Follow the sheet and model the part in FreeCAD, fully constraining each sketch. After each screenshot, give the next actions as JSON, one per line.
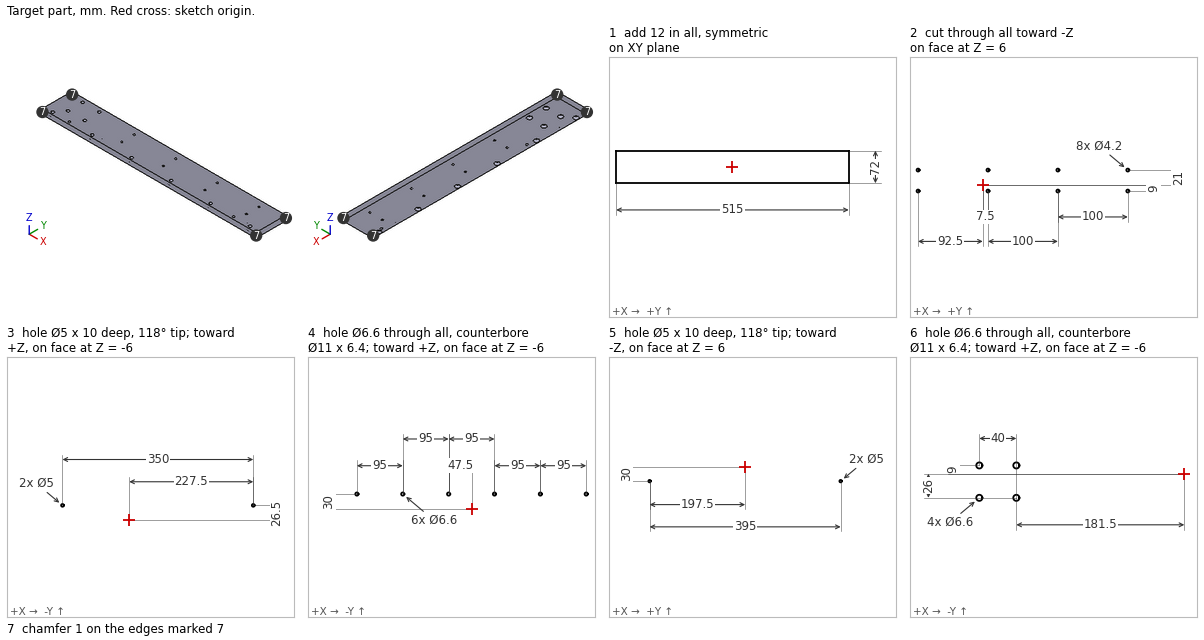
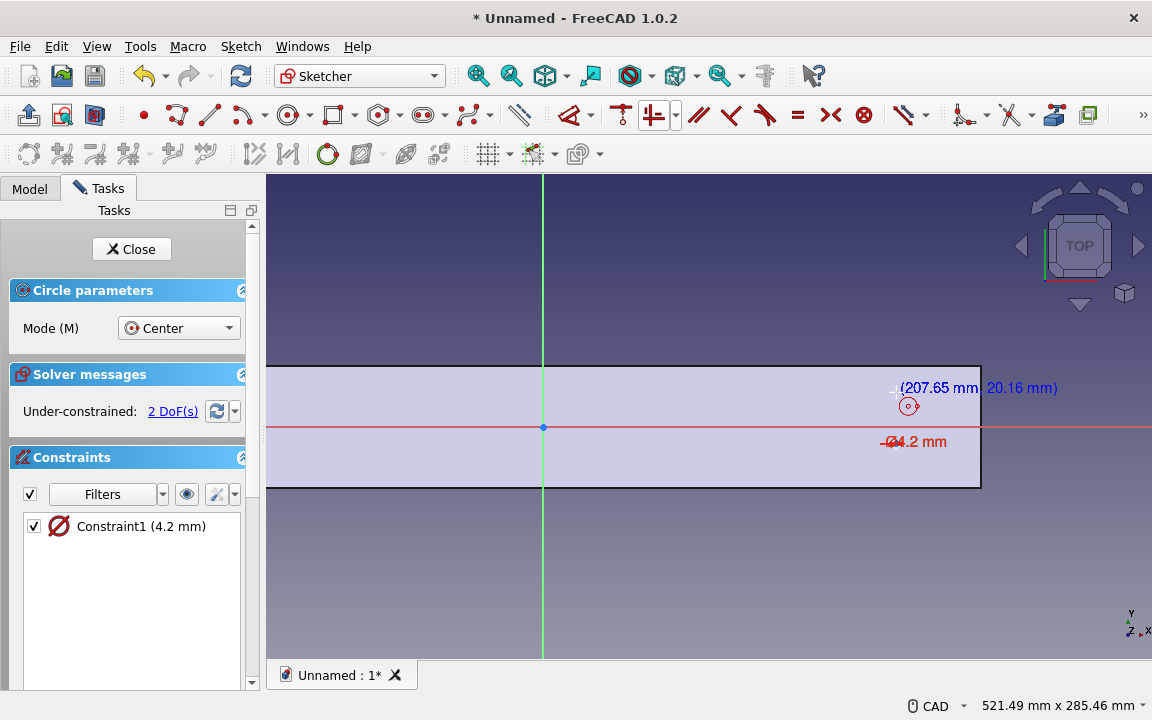
{"action": "left_click", "coordinate": [896, 392]}
{"action": "mouse_move", "coordinate": [898, 389]}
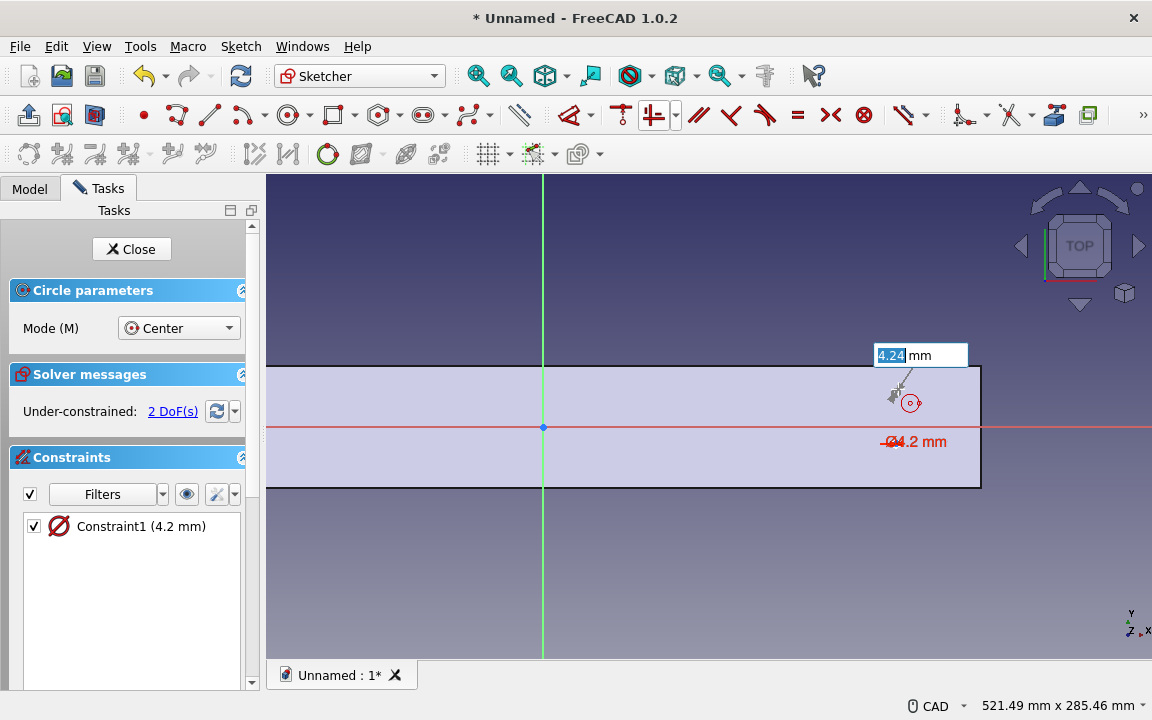
{"action": "type", "text": "4.2"}
{"action": "key", "text": "Return"}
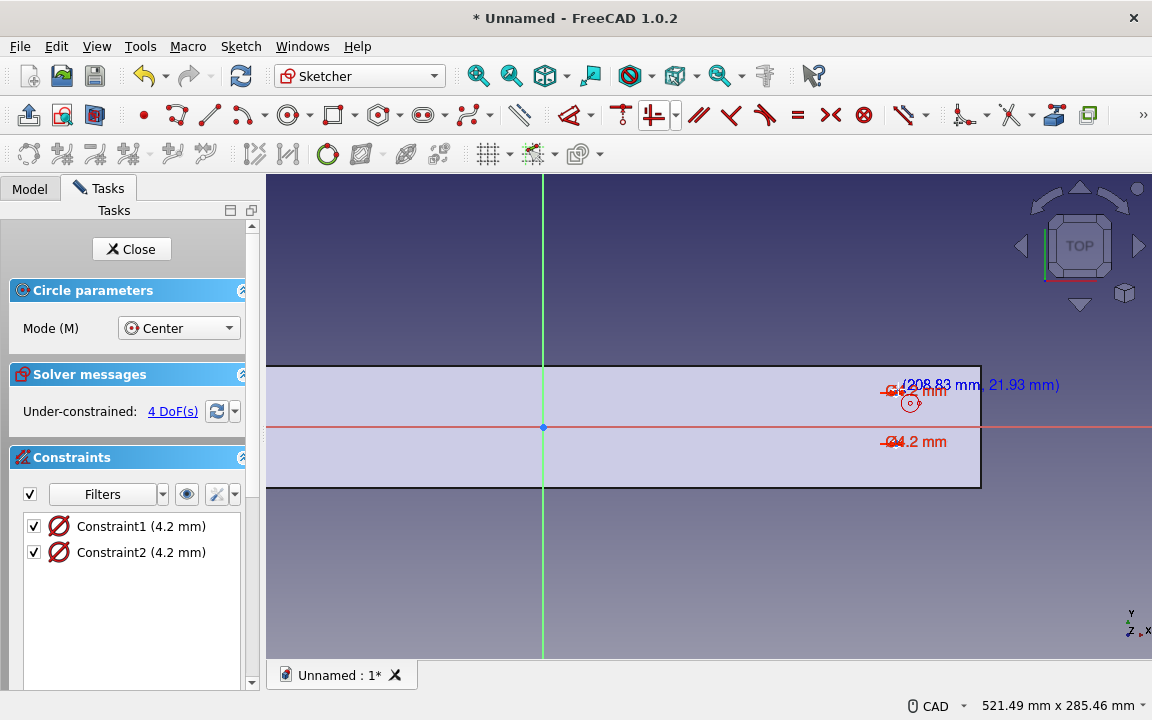
{"action": "scroll", "coordinate": [726, 443], "scroll_direction": "up", "scroll_amount": 10}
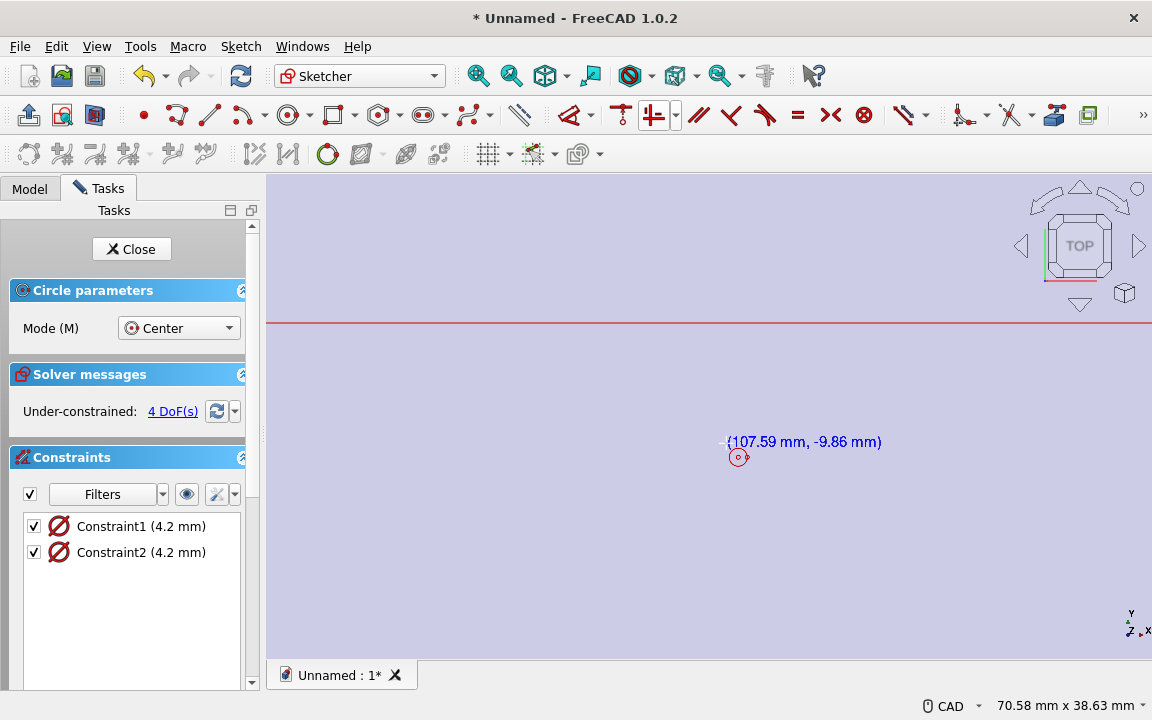
{"action": "scroll", "coordinate": [726, 443], "scroll_direction": "down", "scroll_amount": 10}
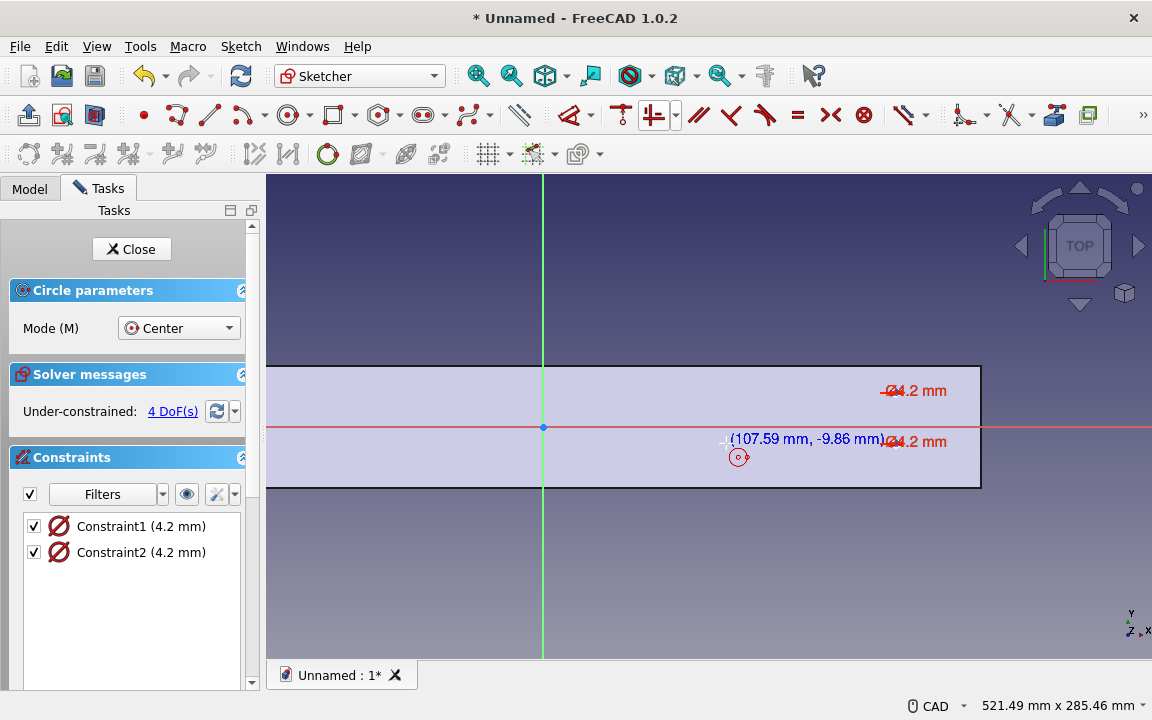
{"action": "left_click", "coordinate": [726, 443]}
{"action": "mouse_move", "coordinate": [728, 445]}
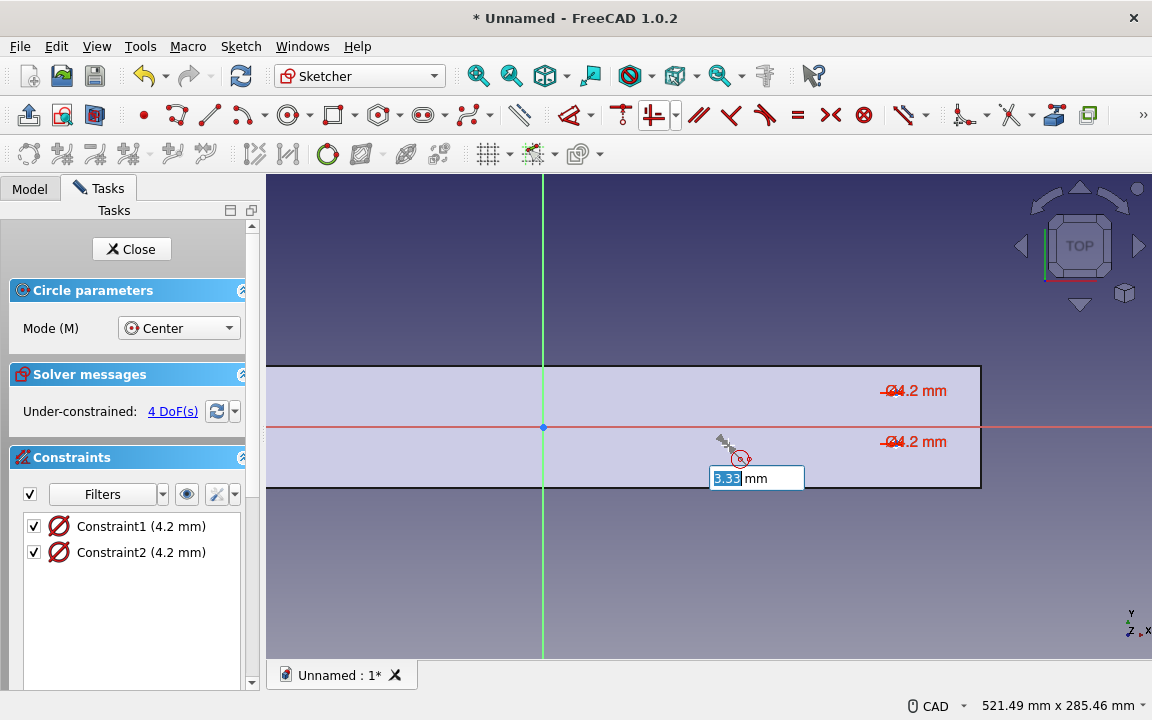
{"action": "type", "text": "4.2"}
{"action": "key", "text": "Return"}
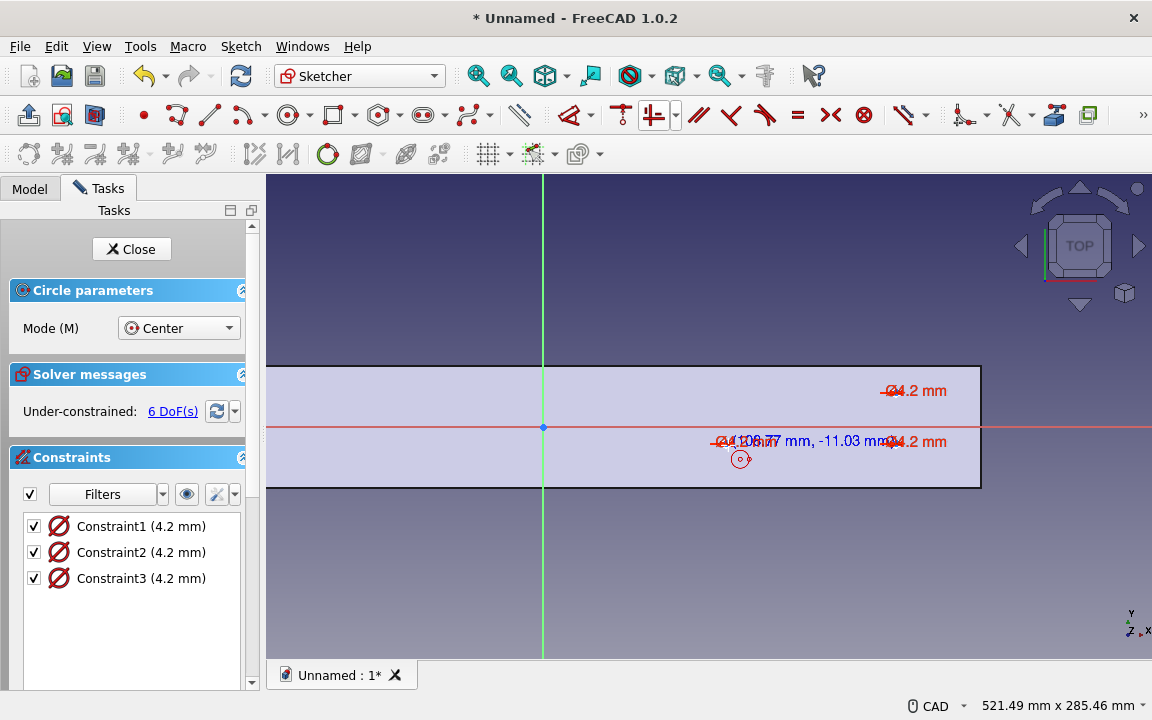
{"action": "scroll", "coordinate": [726, 392], "scroll_direction": "up", "scroll_amount": 10}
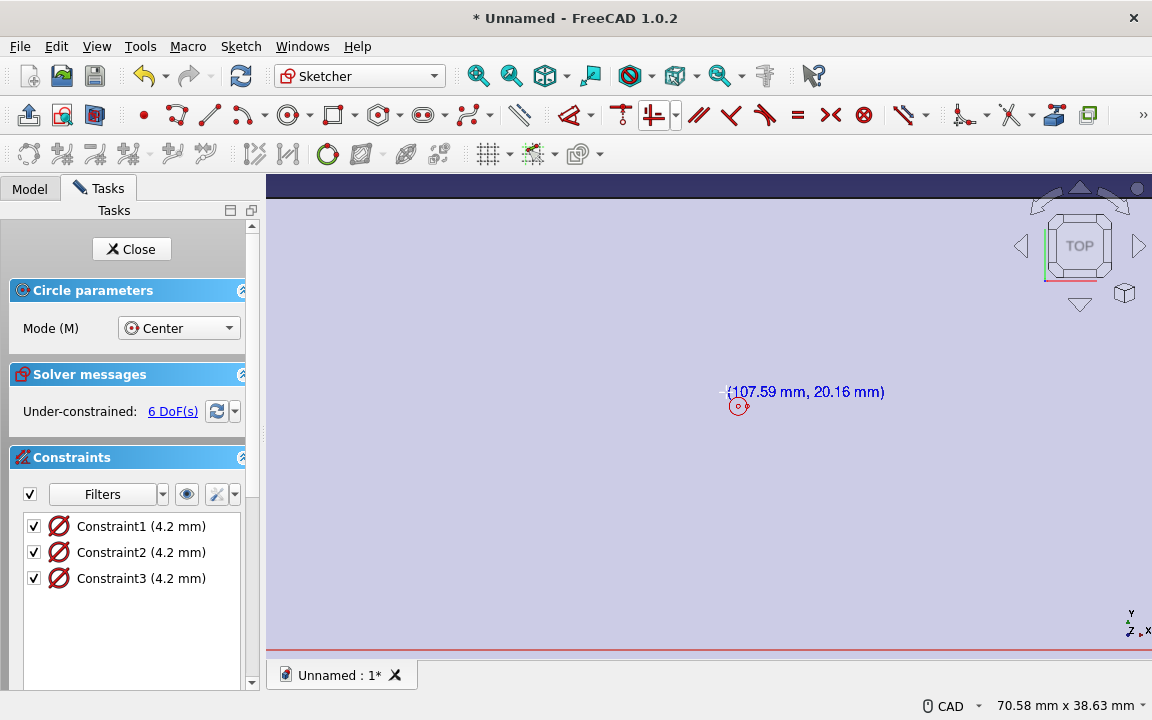
{"action": "scroll", "coordinate": [726, 392], "scroll_direction": "down", "scroll_amount": 10}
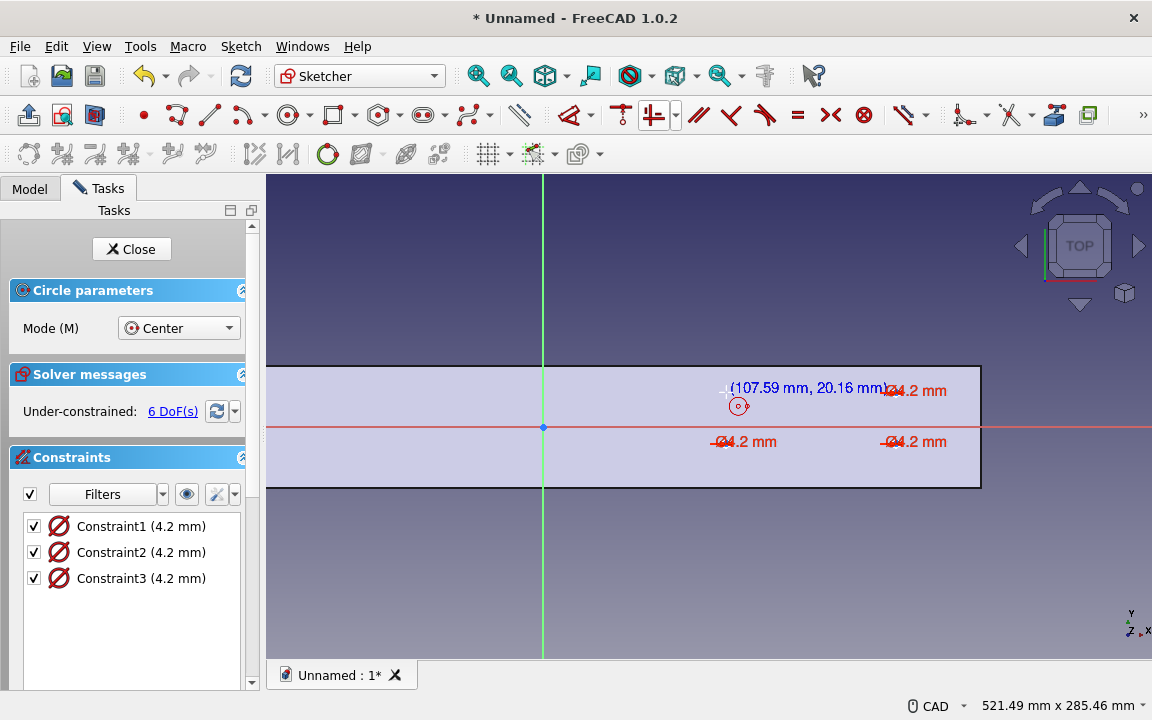
{"action": "left_click", "coordinate": [726, 392]}
{"action": "mouse_move", "coordinate": [728, 389]}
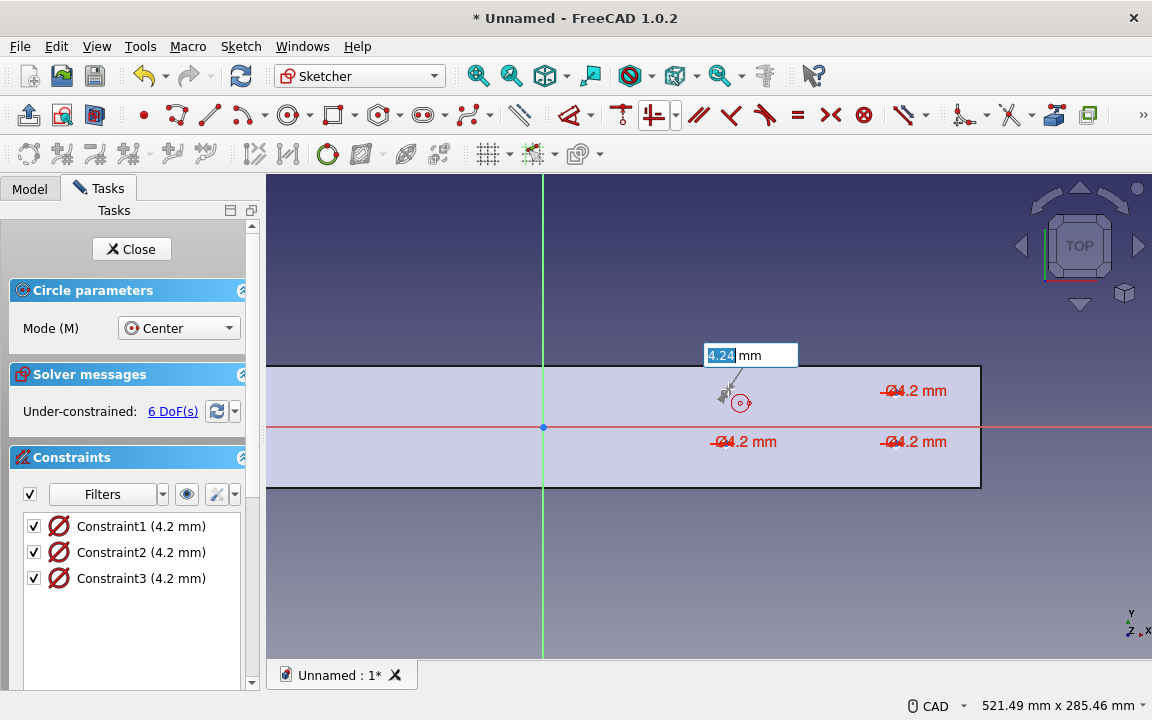
{"action": "type", "text": "4.2"}
{"action": "key", "text": "Return"}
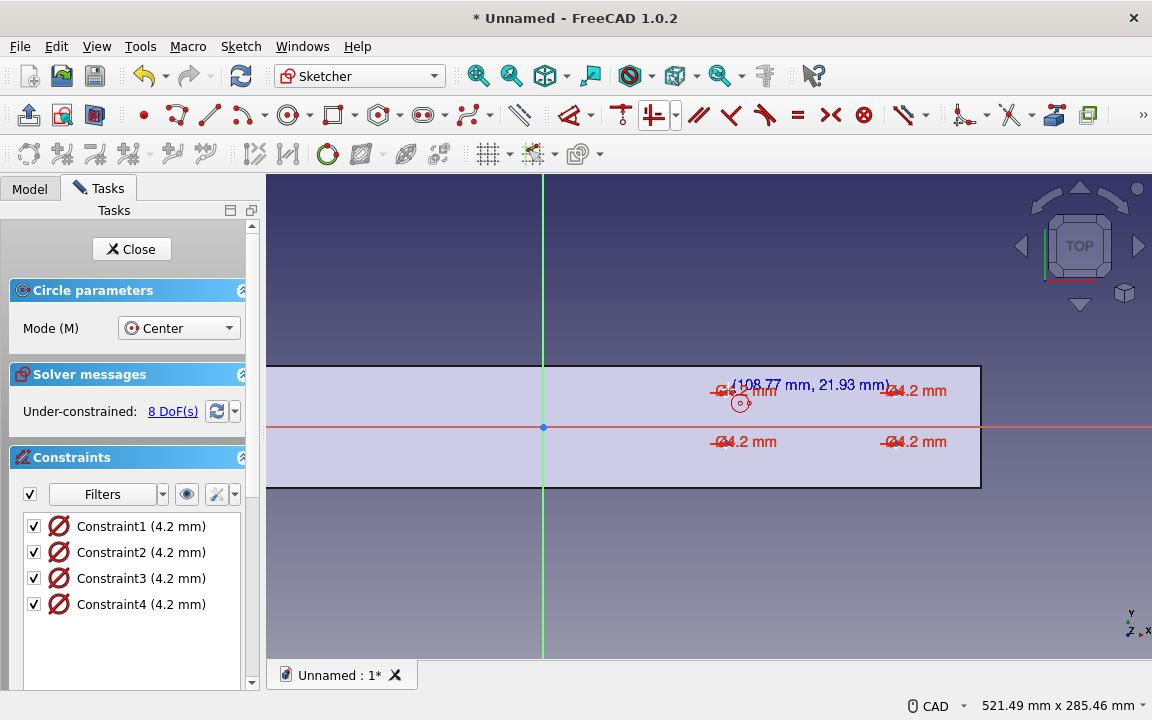
{"action": "scroll", "coordinate": [556, 443], "scroll_direction": "up", "scroll_amount": 10}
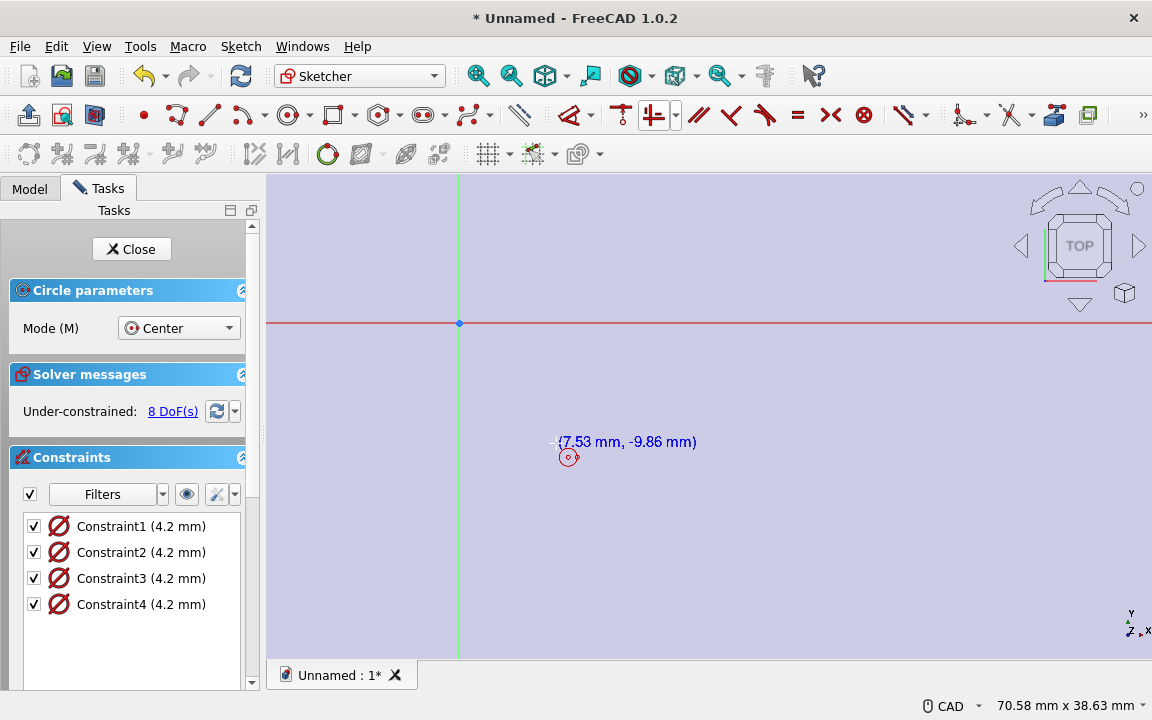
{"action": "scroll", "coordinate": [556, 443], "scroll_direction": "down", "scroll_amount": 10}